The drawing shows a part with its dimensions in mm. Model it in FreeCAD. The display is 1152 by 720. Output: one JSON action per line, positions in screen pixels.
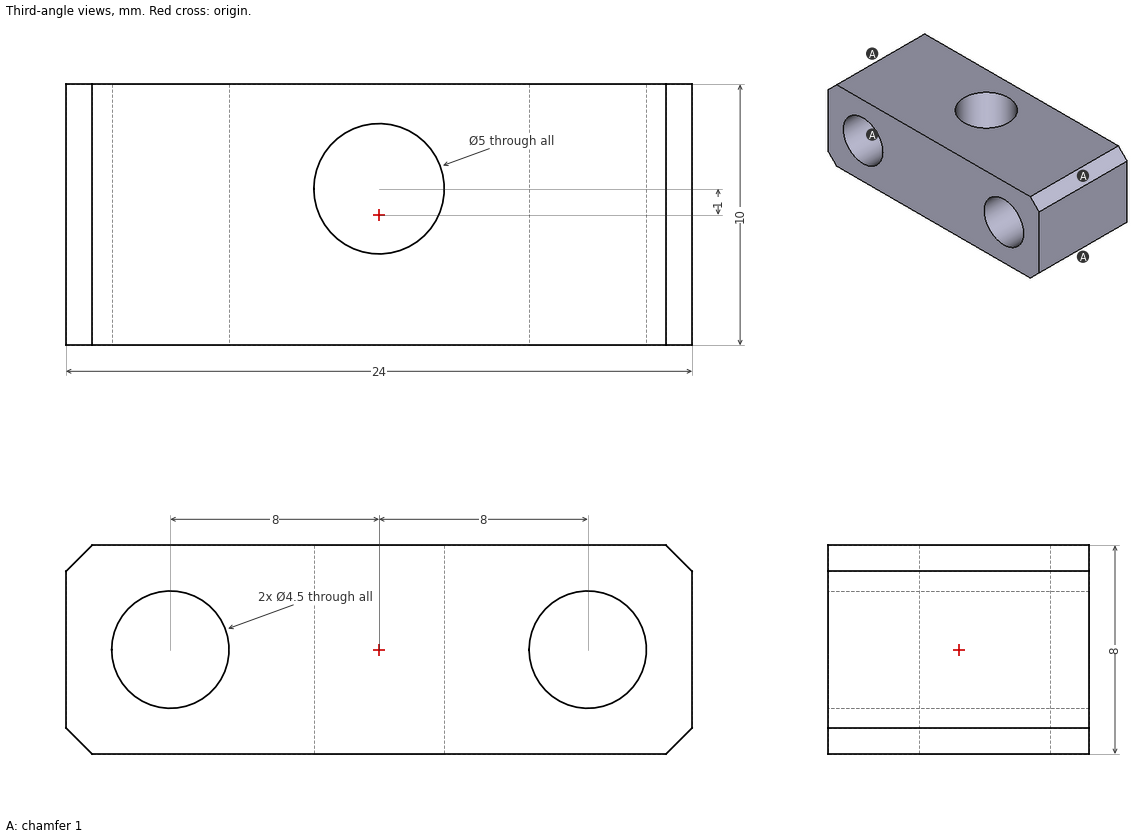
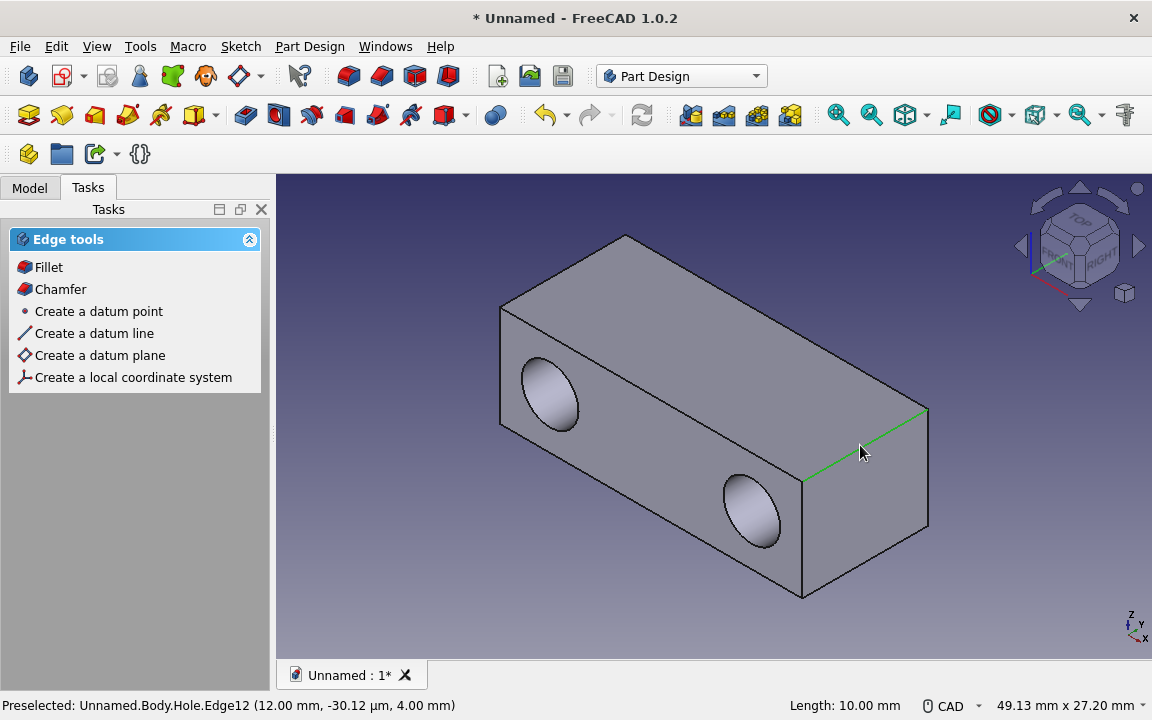
{"action": "key", "text": "2"}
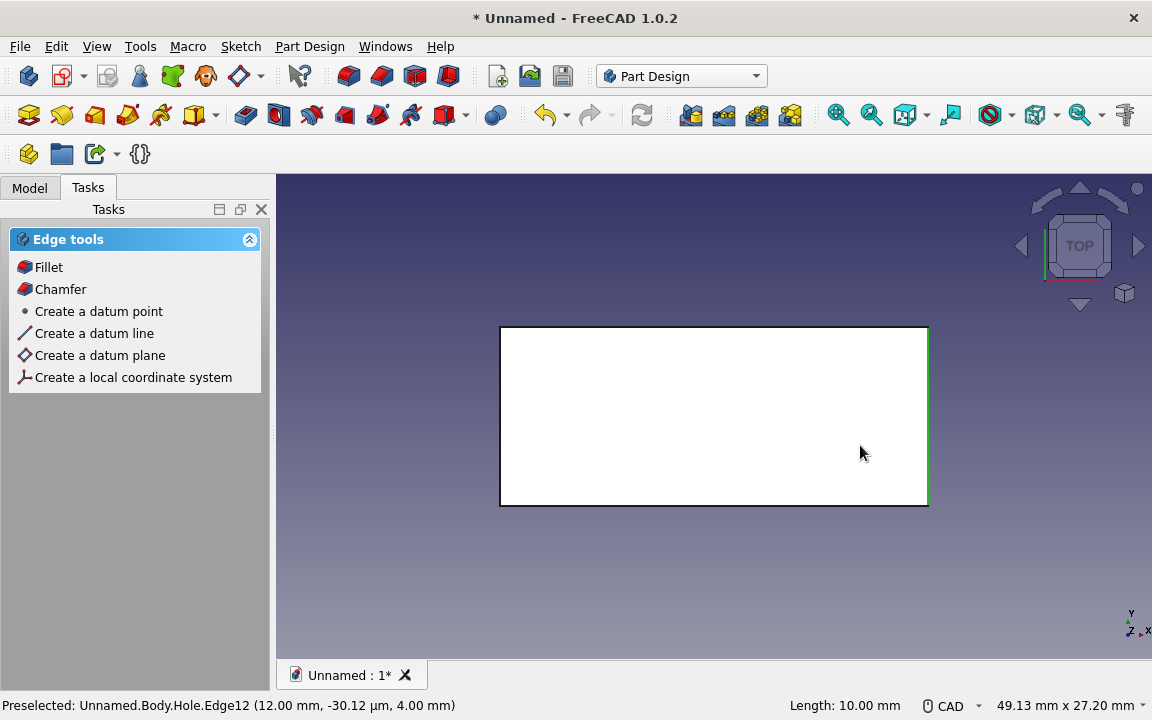
{"action": "left_click", "coordinate": [500, 415], "text": "ctrl"}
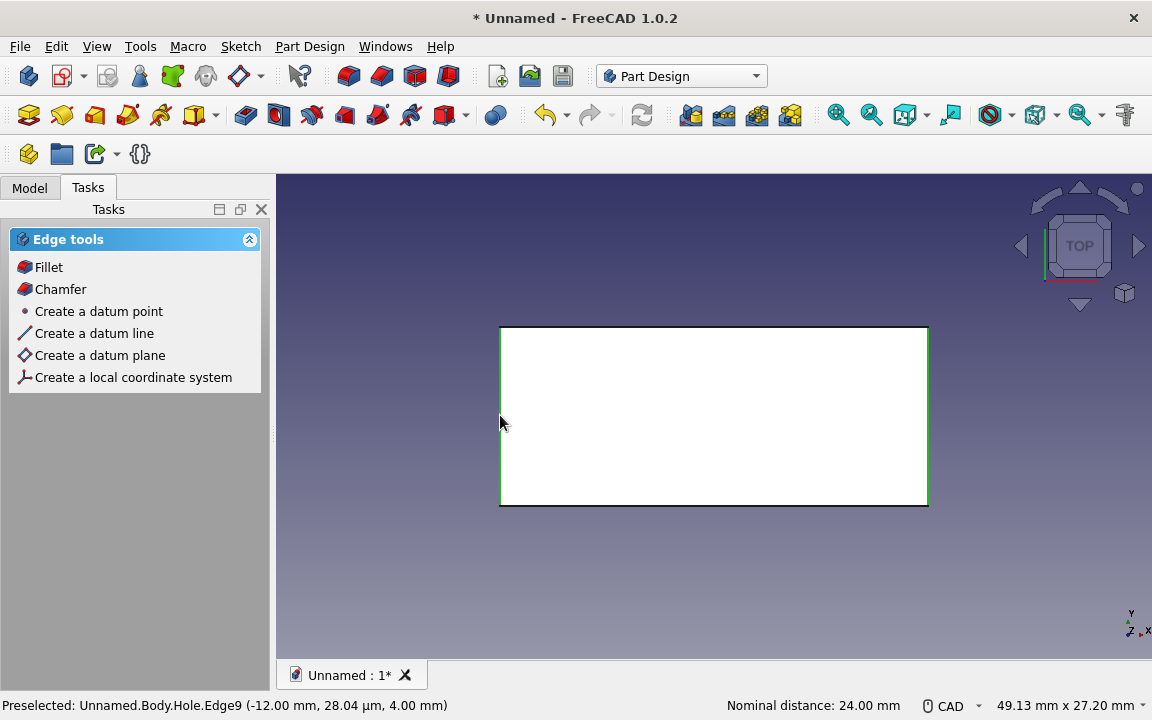
{"action": "key", "text": "1"}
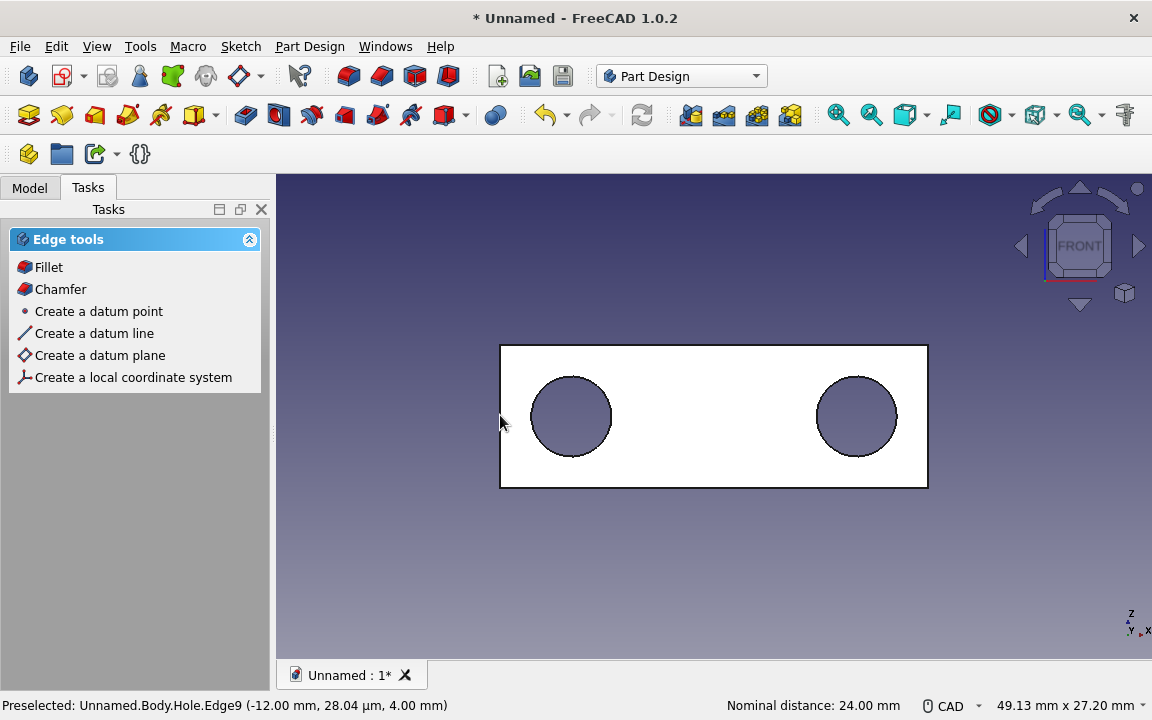
{"action": "key", "text": "3"}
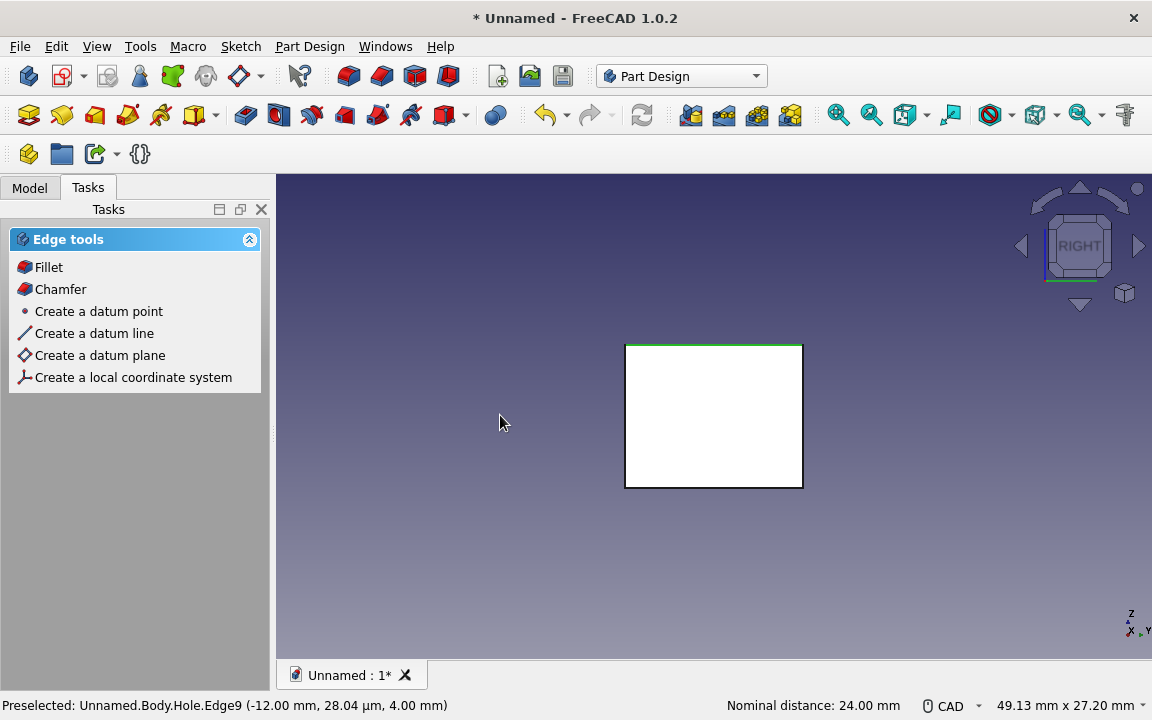
{"action": "left_click", "coordinate": [839, 116]}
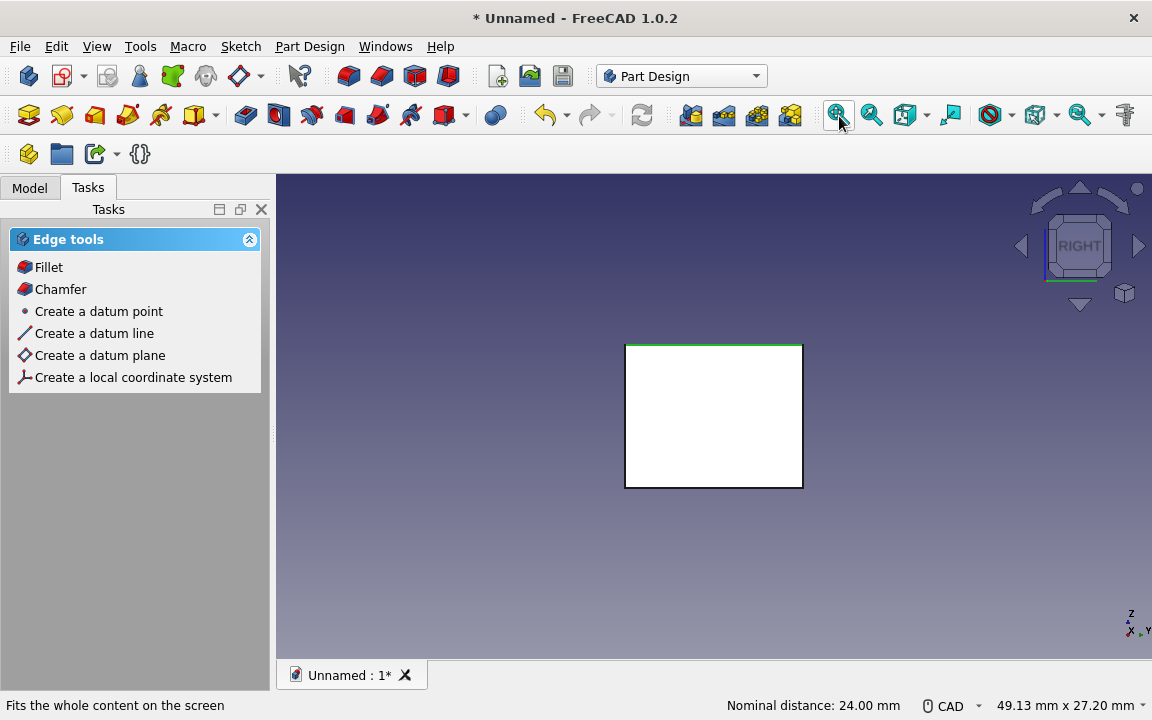
{"action": "left_click", "coordinate": [714, 487], "text": "ctrl"}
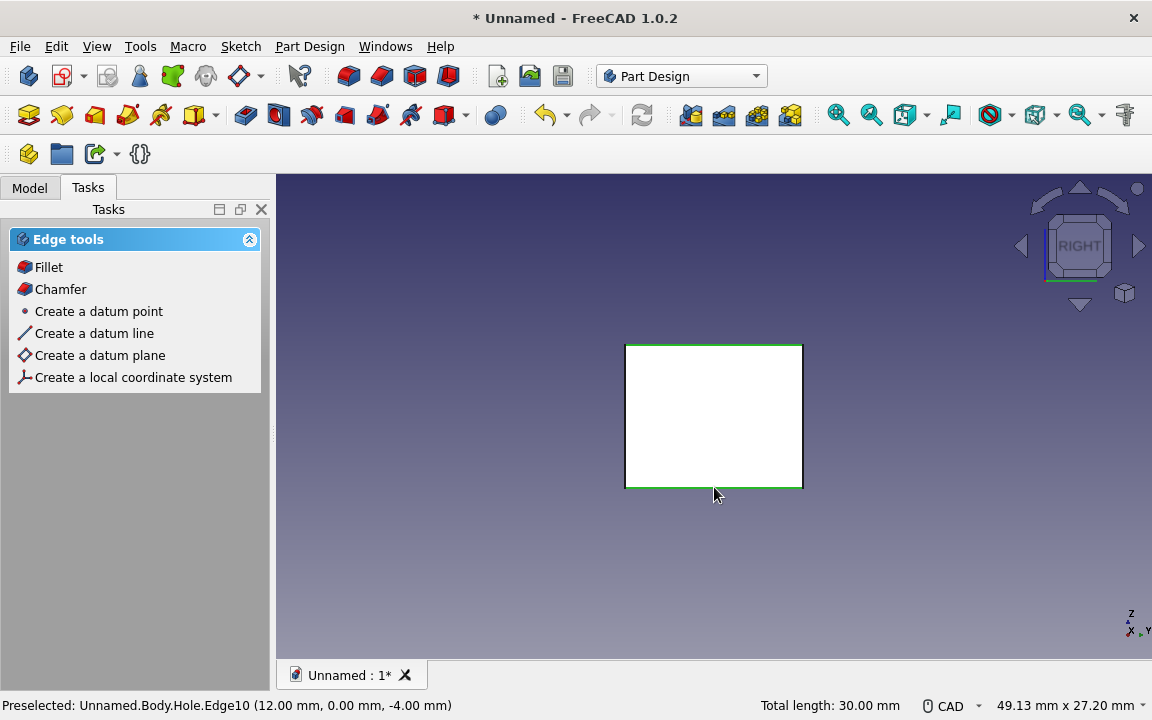
{"action": "key", "text": "5"}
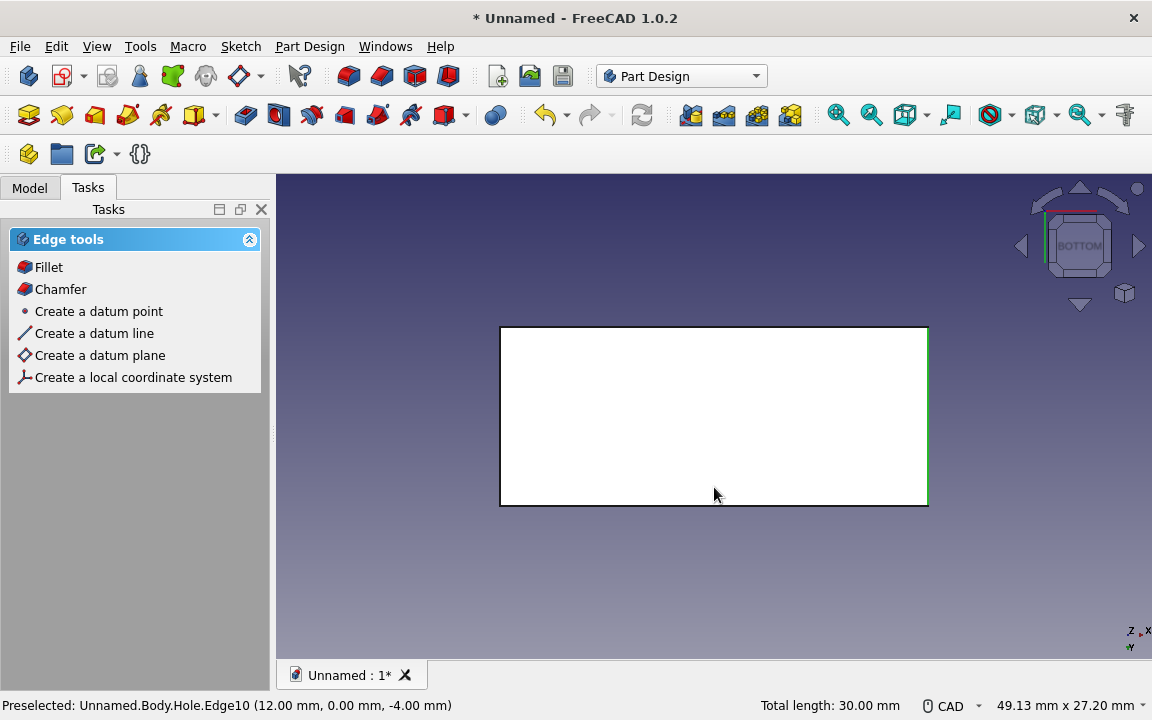
{"action": "left_click", "coordinate": [500, 415], "text": "ctrl"}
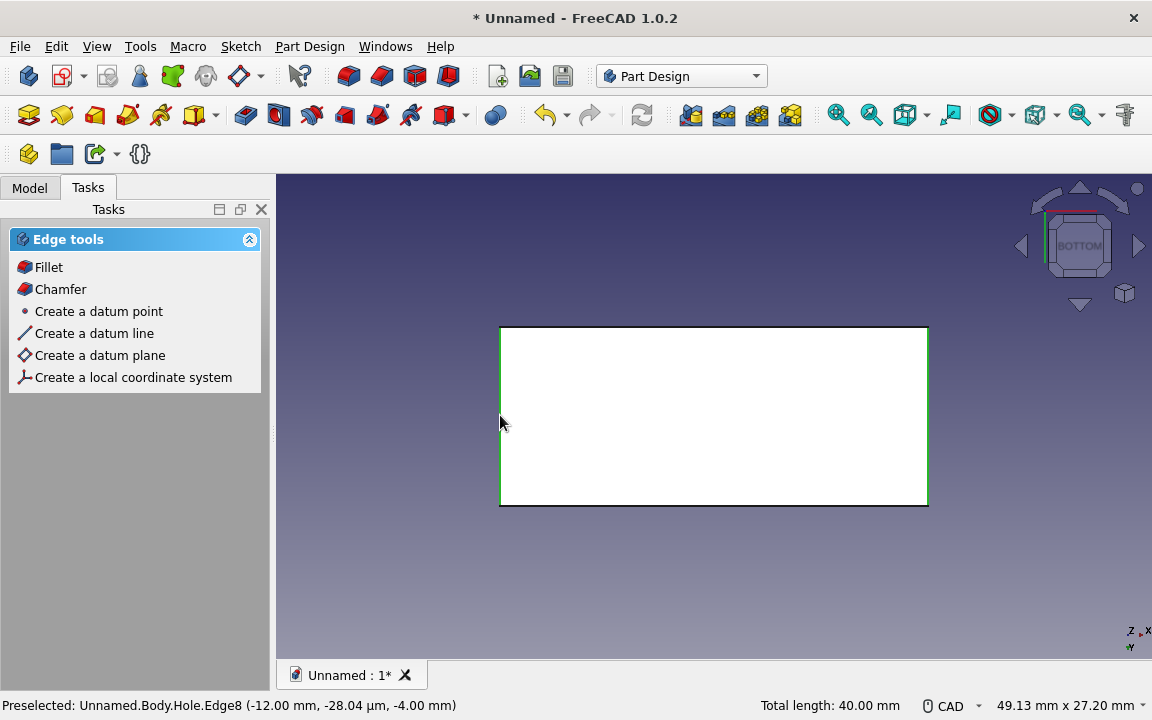
{"action": "left_click", "coordinate": [382, 76]}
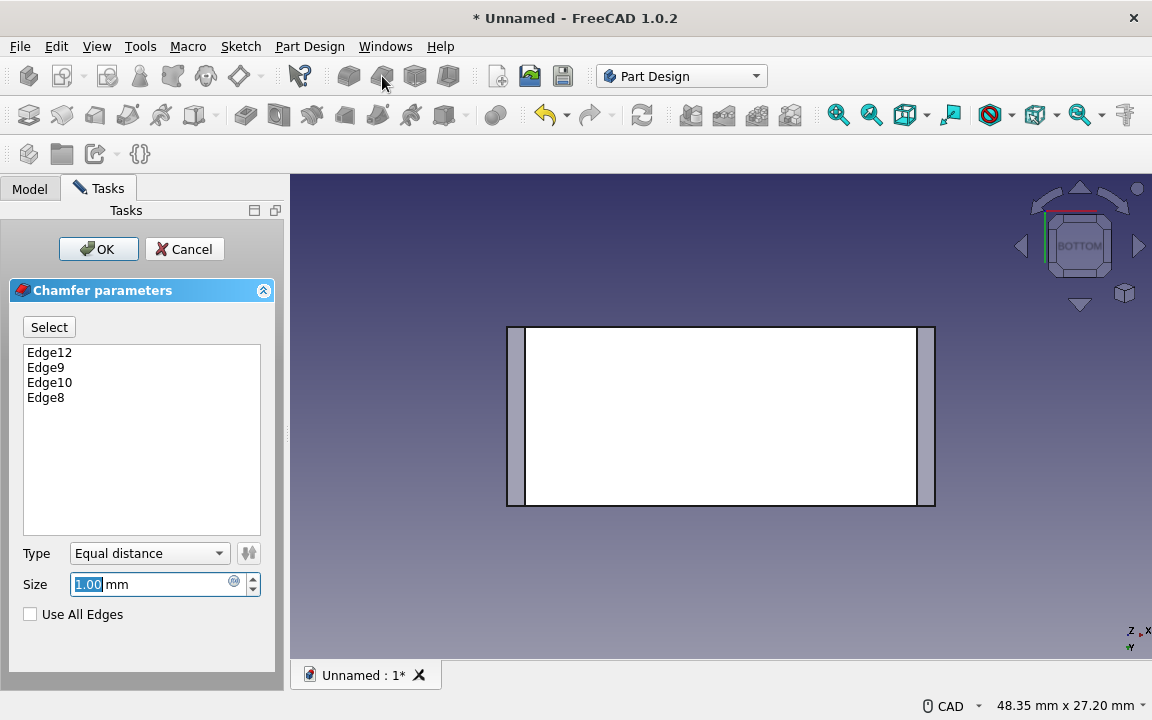
{"action": "type", "text": "1"}
{"action": "key", "text": "Tab"}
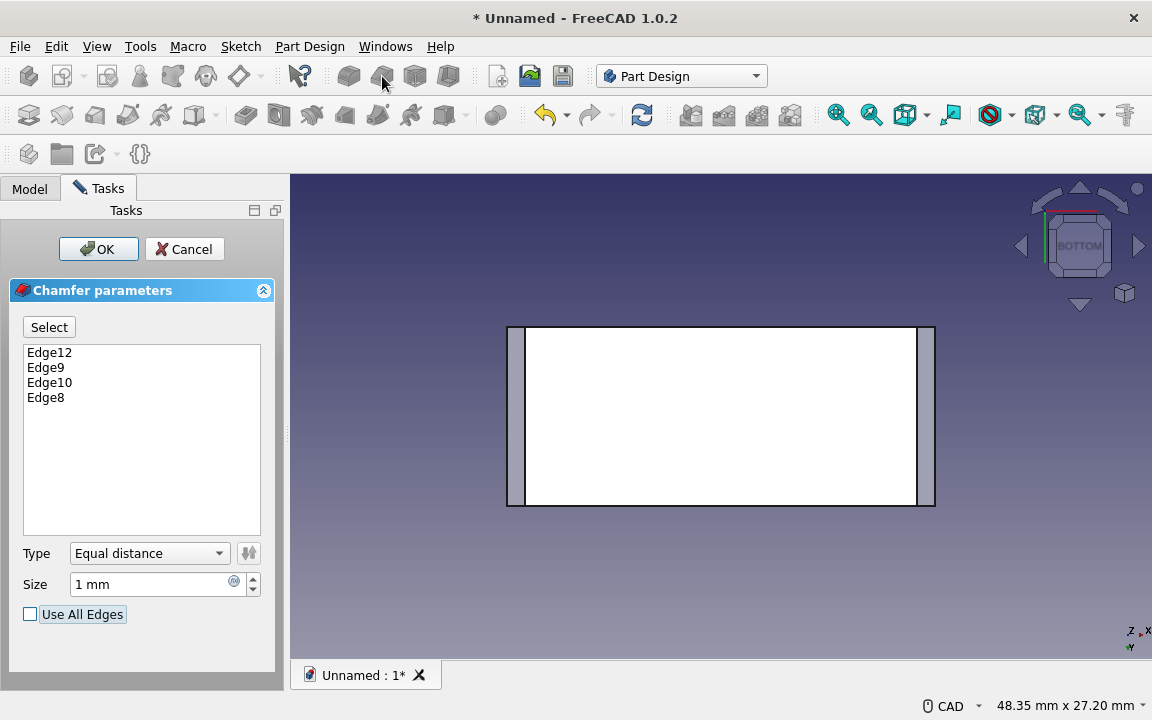
{"action": "left_click", "coordinate": [99, 249]}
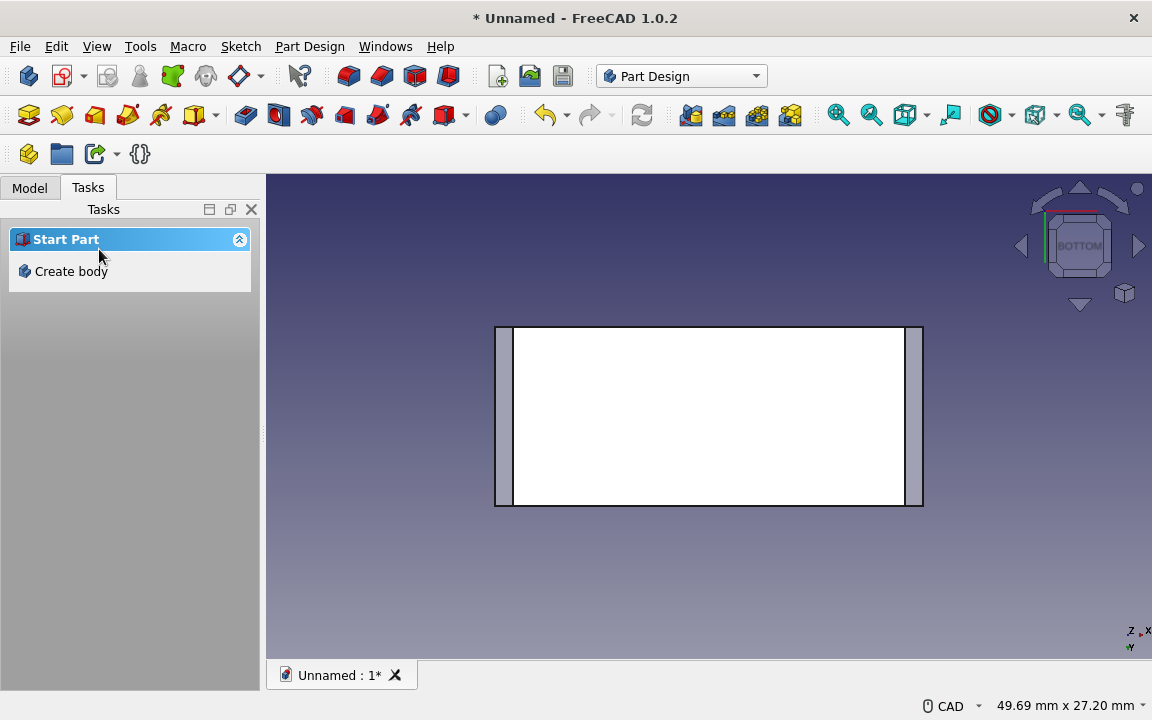
{"action": "key", "text": "0"}